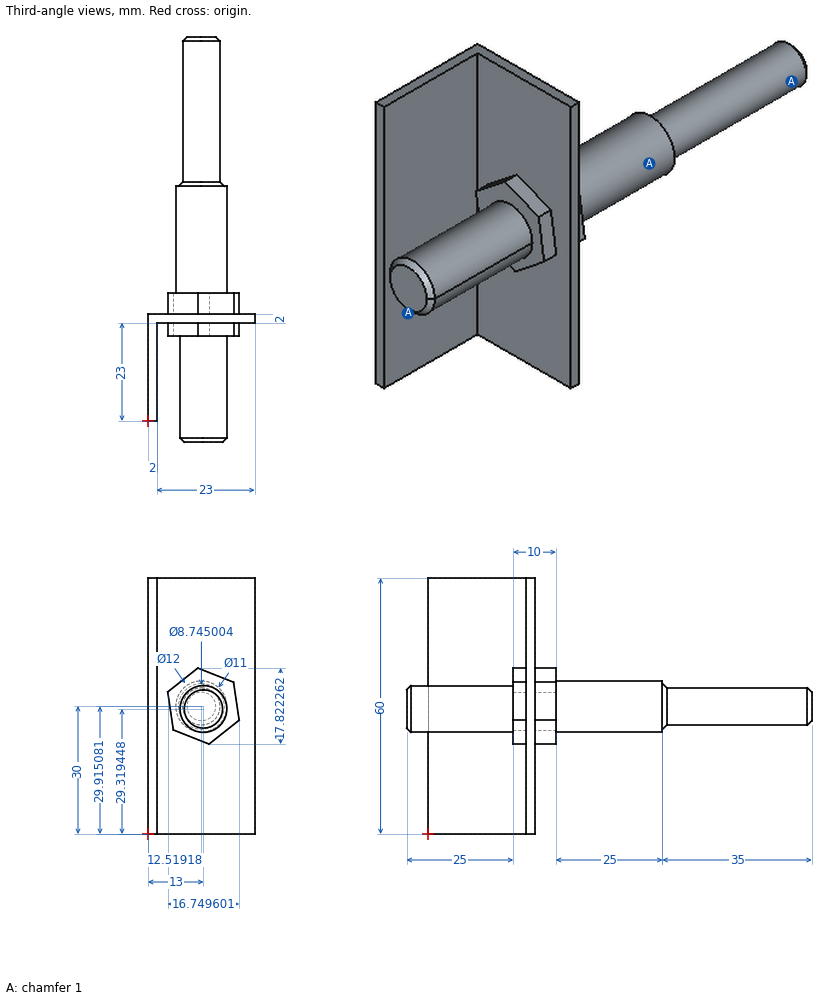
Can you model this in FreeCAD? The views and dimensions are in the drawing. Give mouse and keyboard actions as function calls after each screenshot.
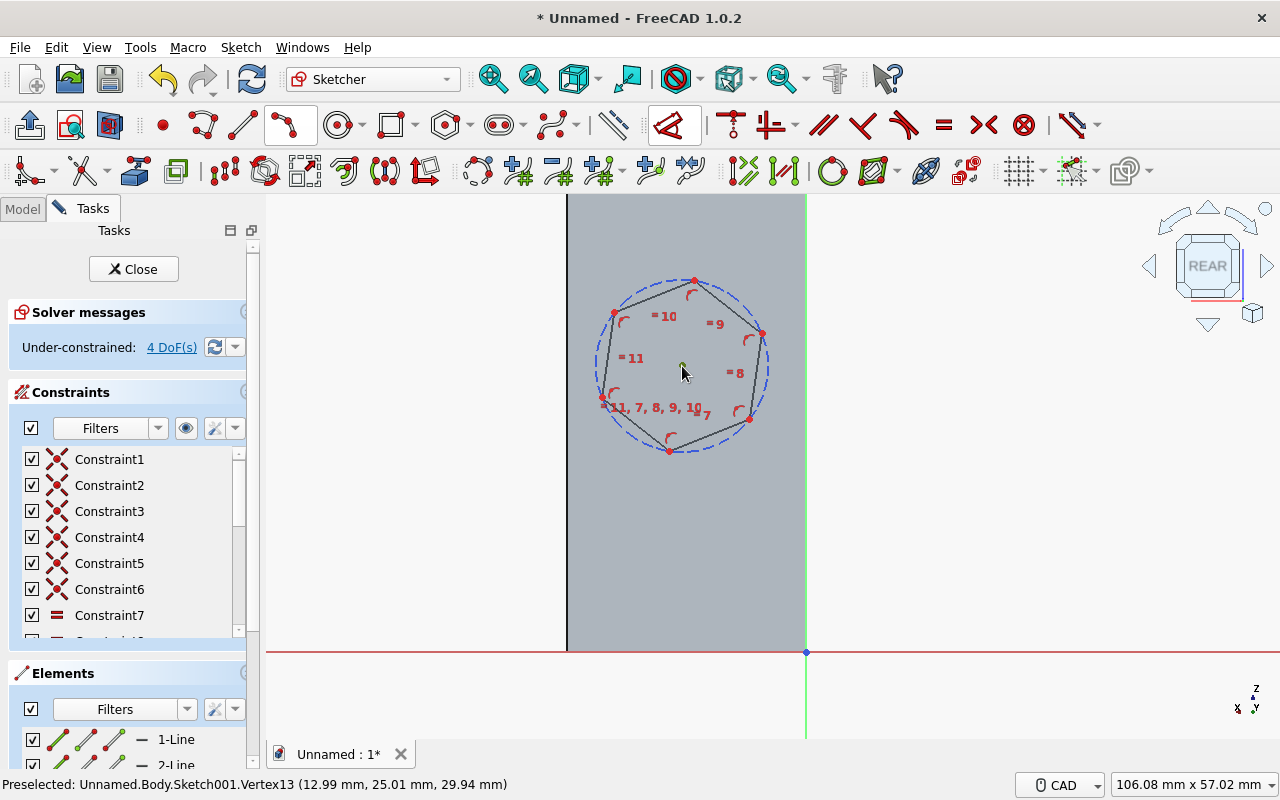
key(l)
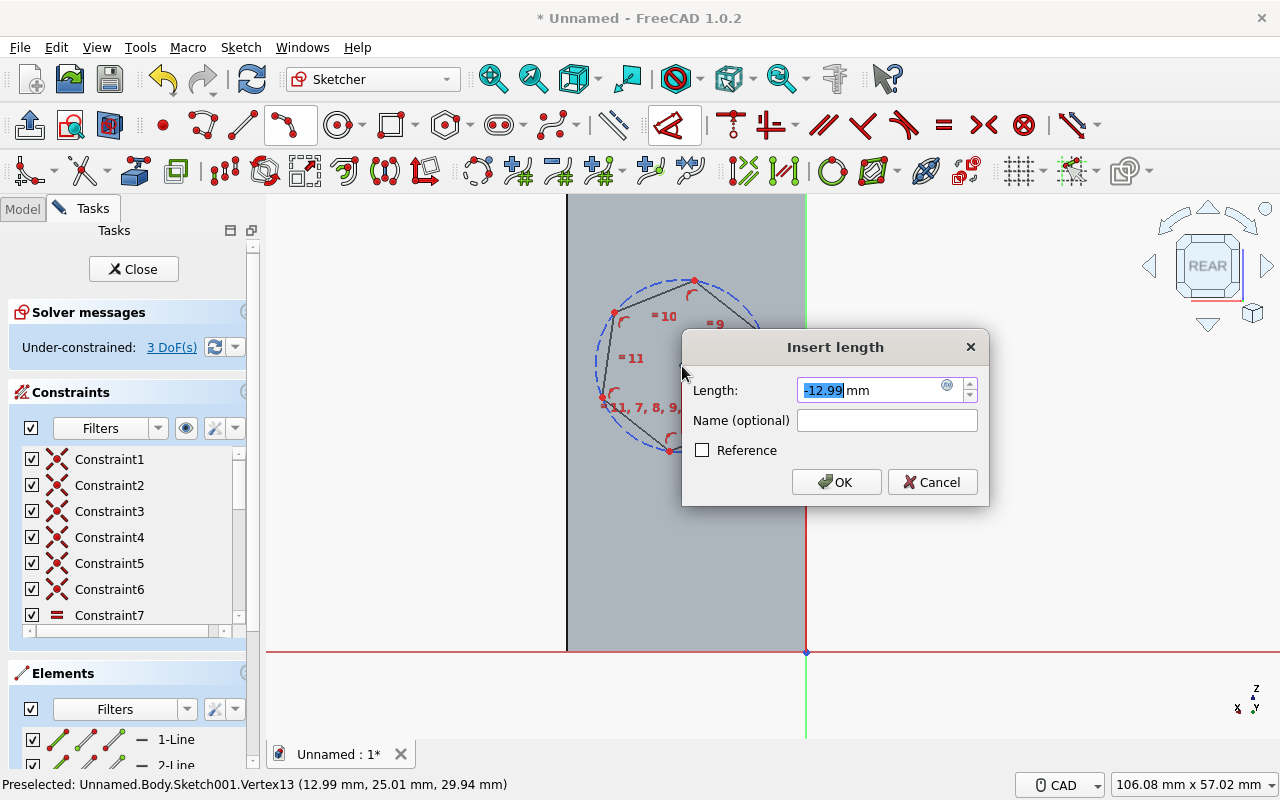
text(-13)
key(Return)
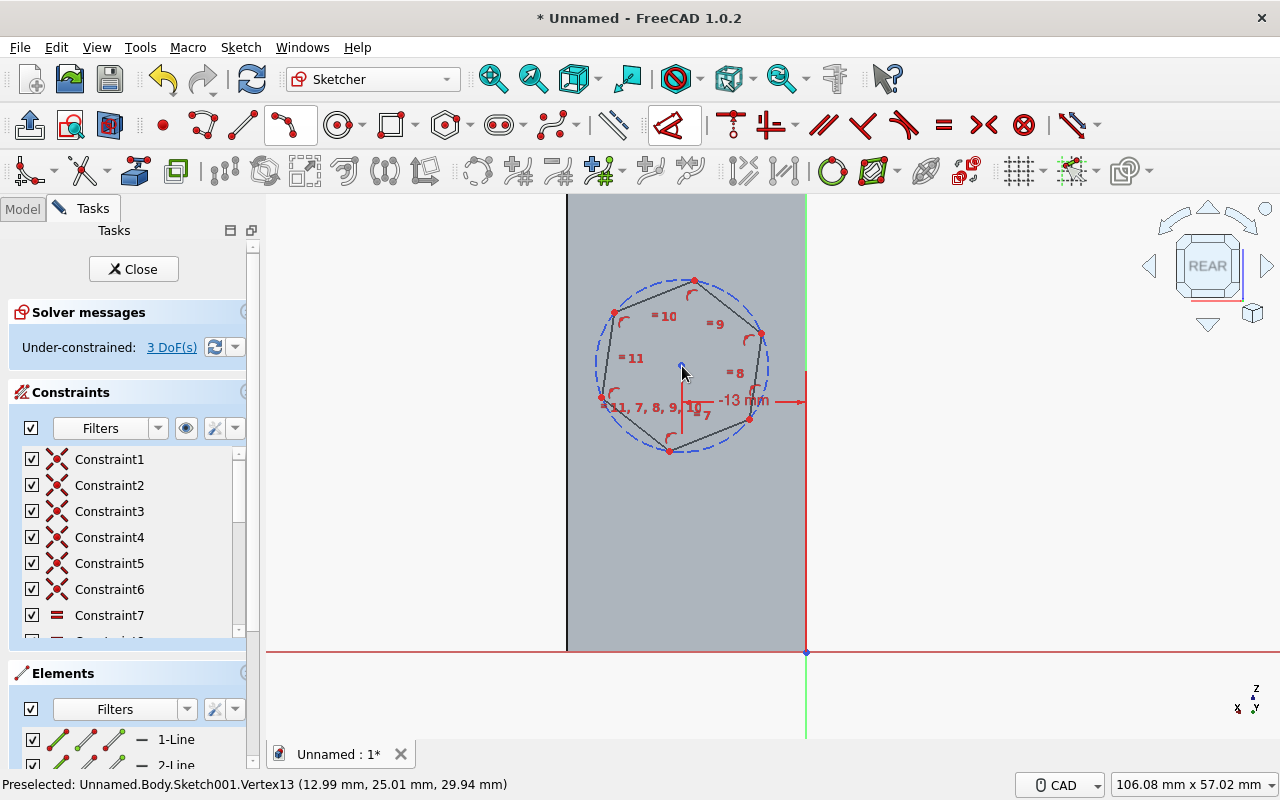
click(682, 366)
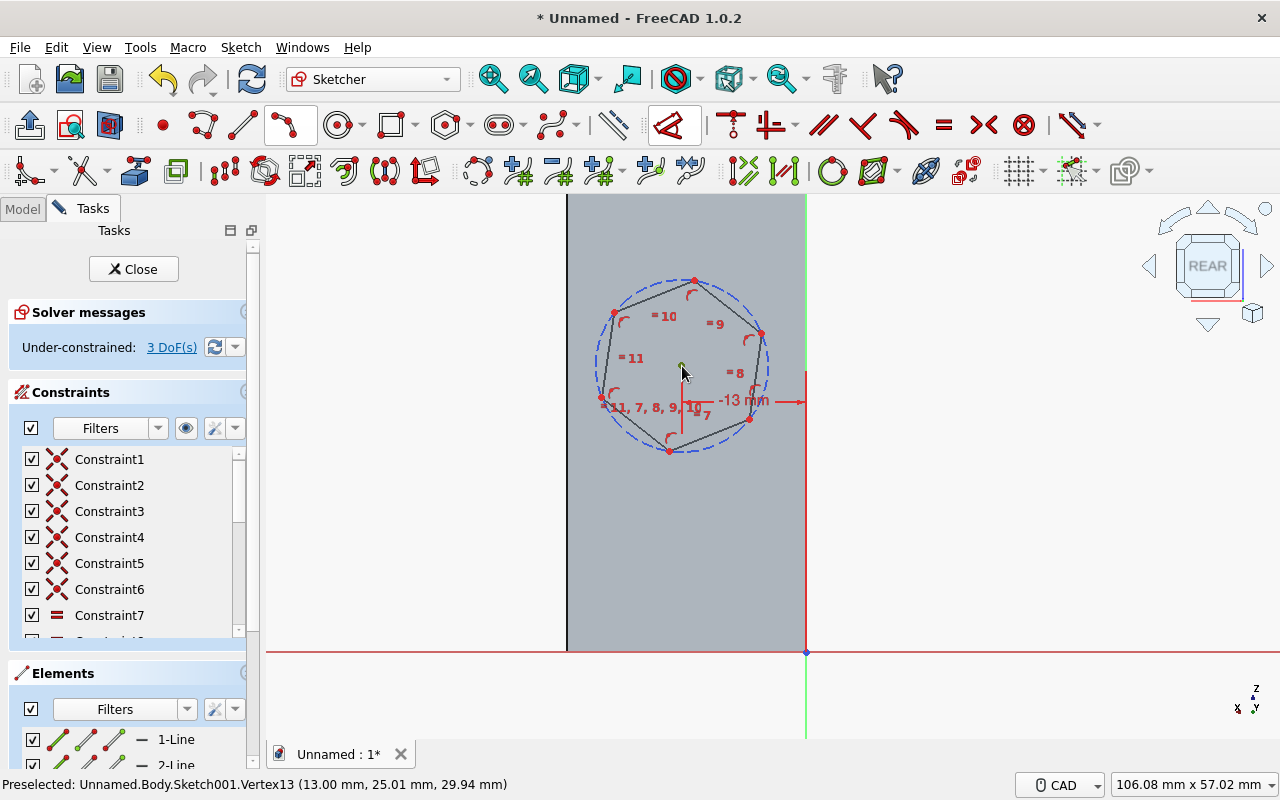
key(i)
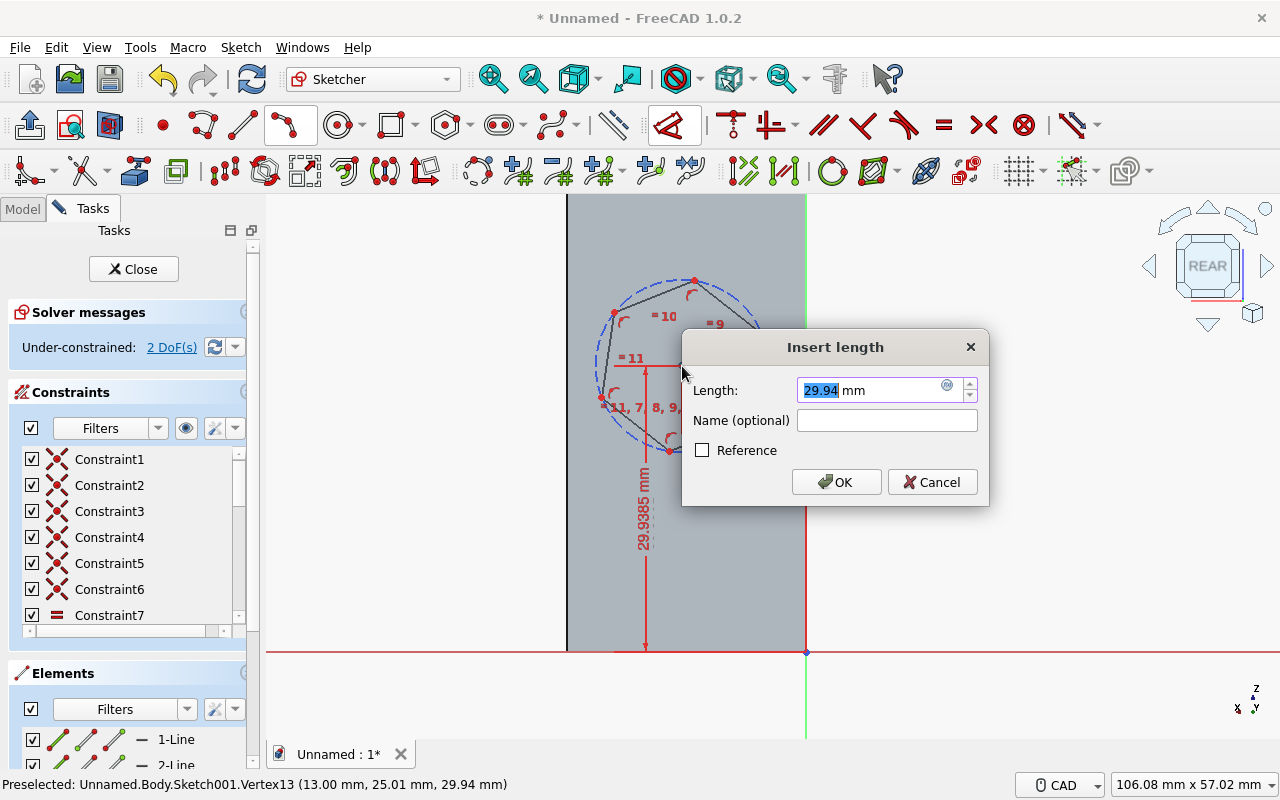
text(30)
key(Return)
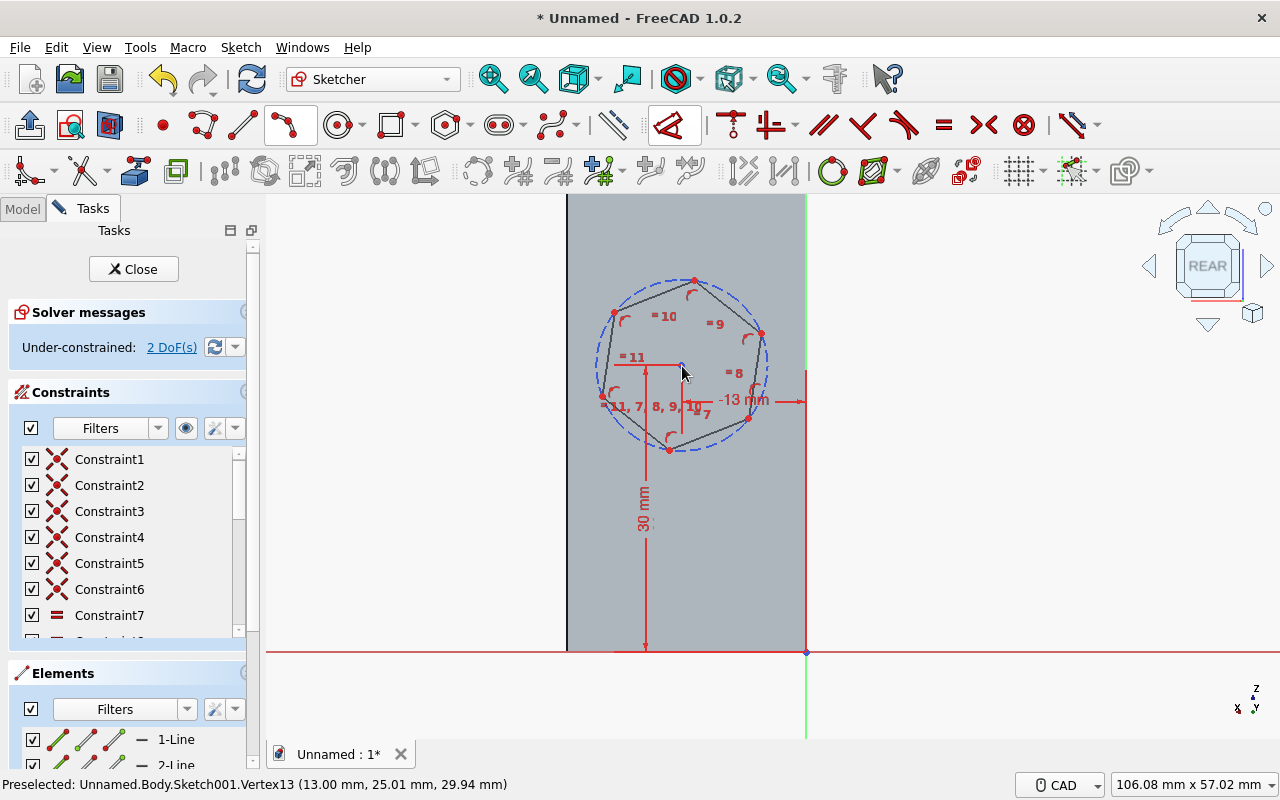
click(602, 397)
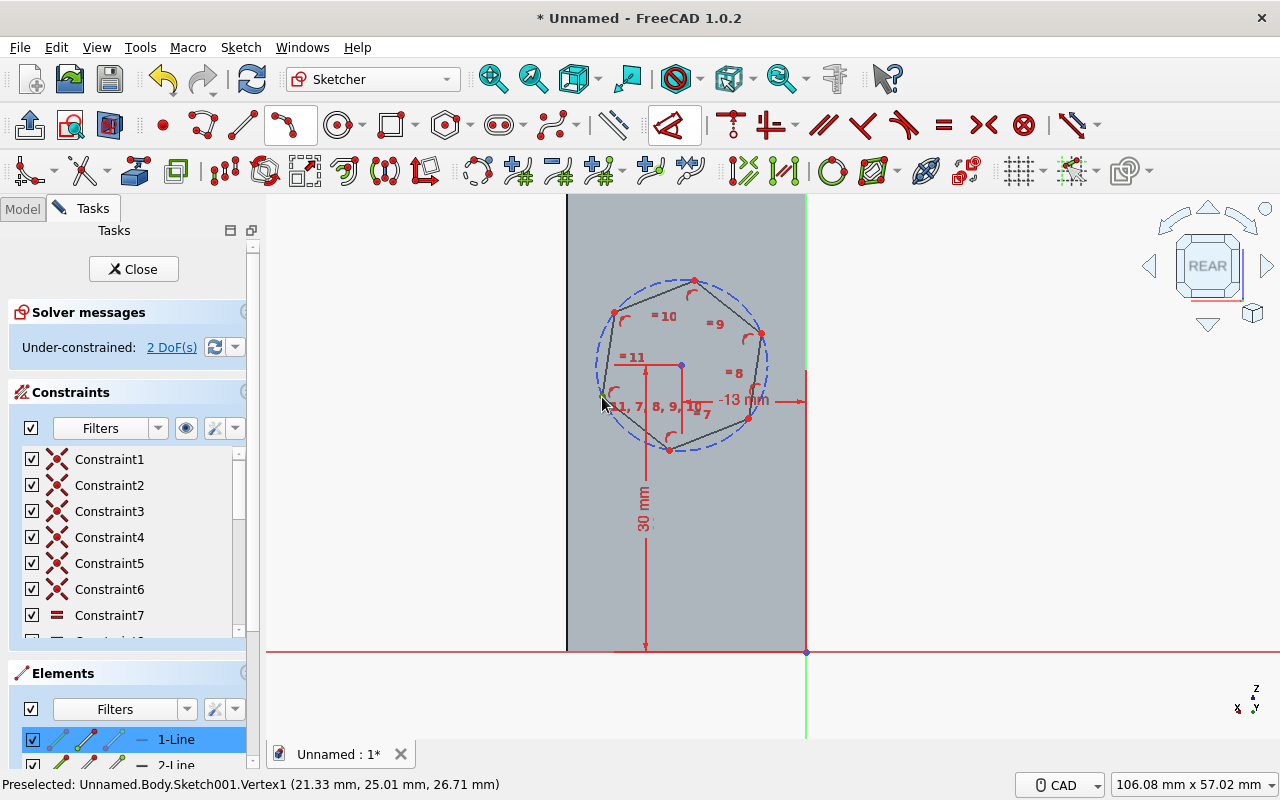
click(762, 334)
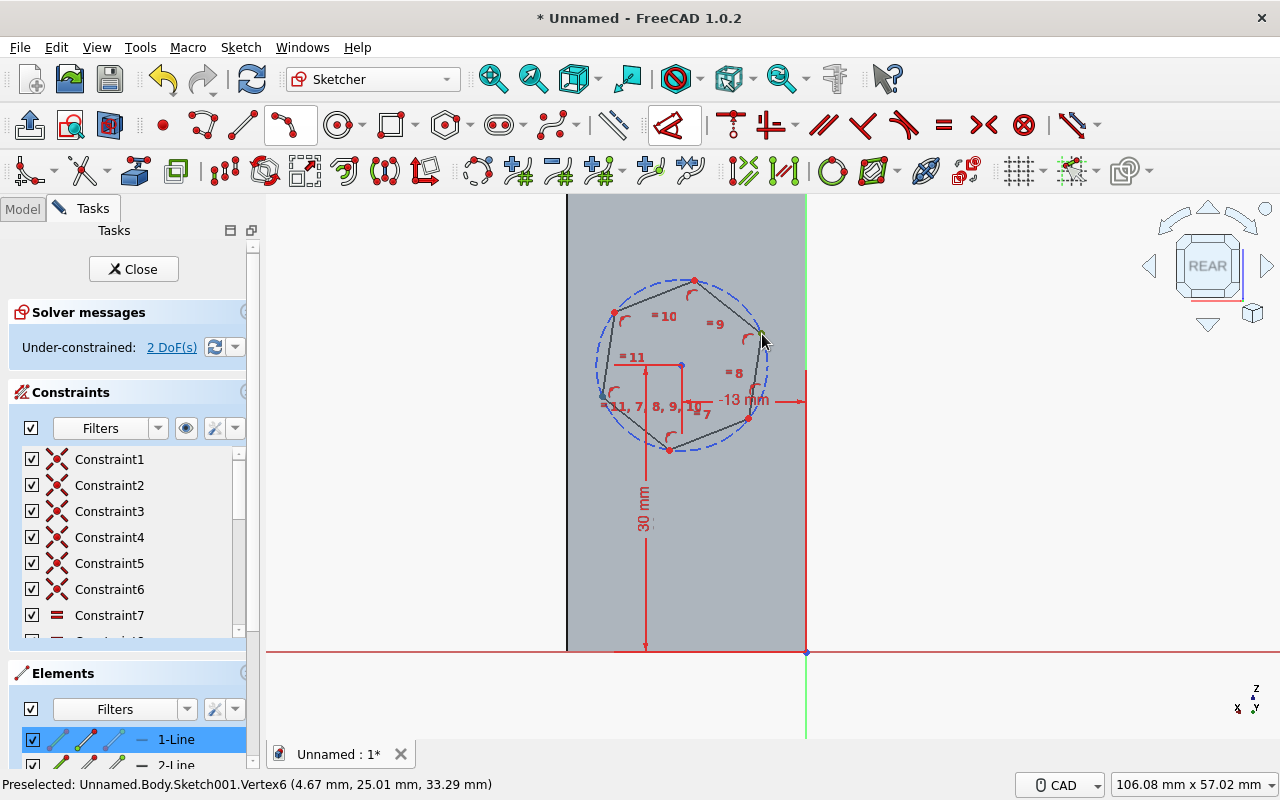
key(l)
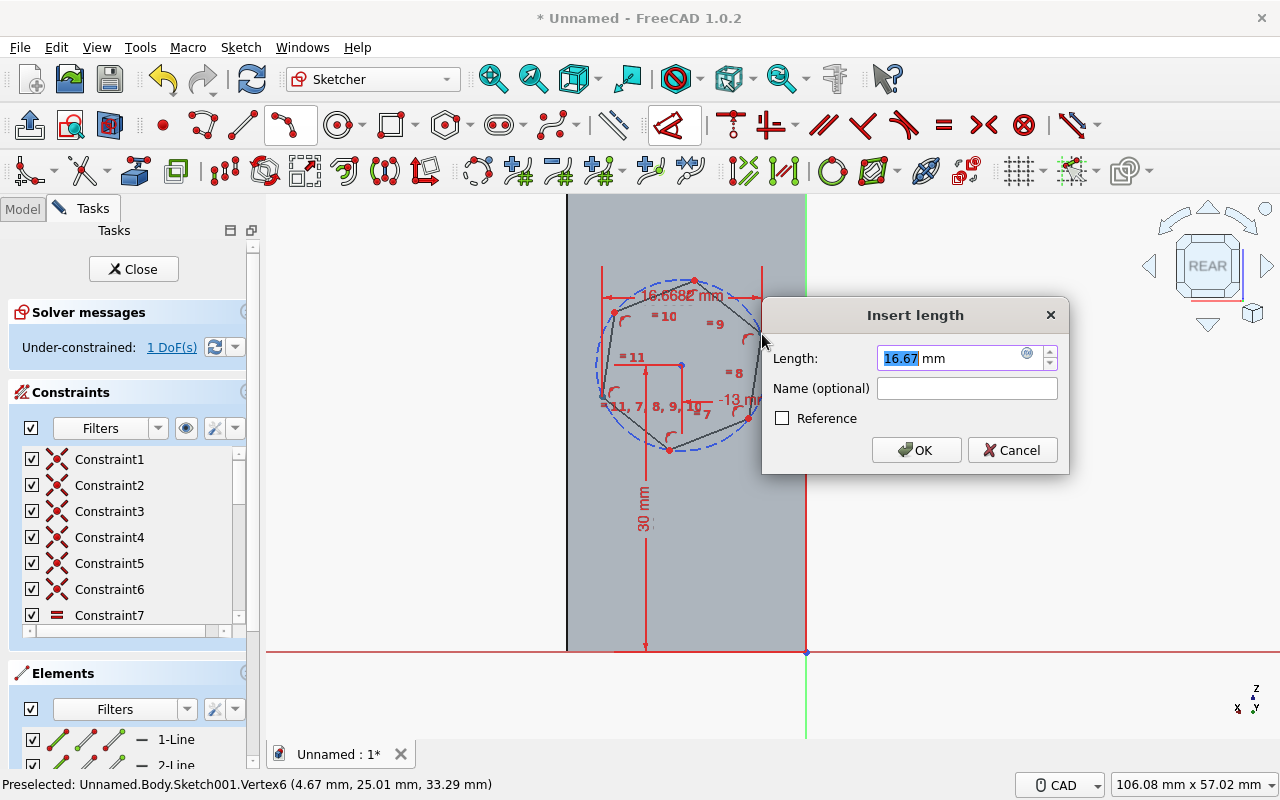
text(16.749601)
key(Return)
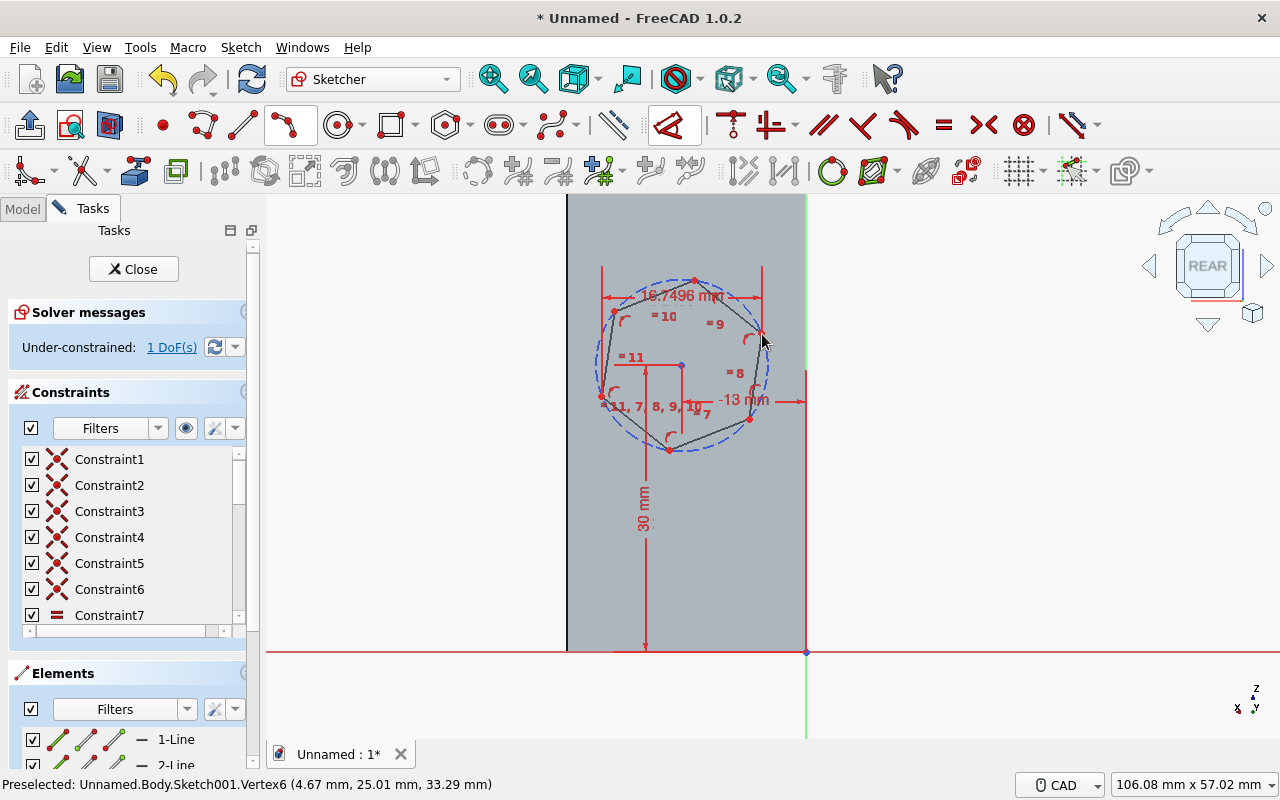
click(669, 450)